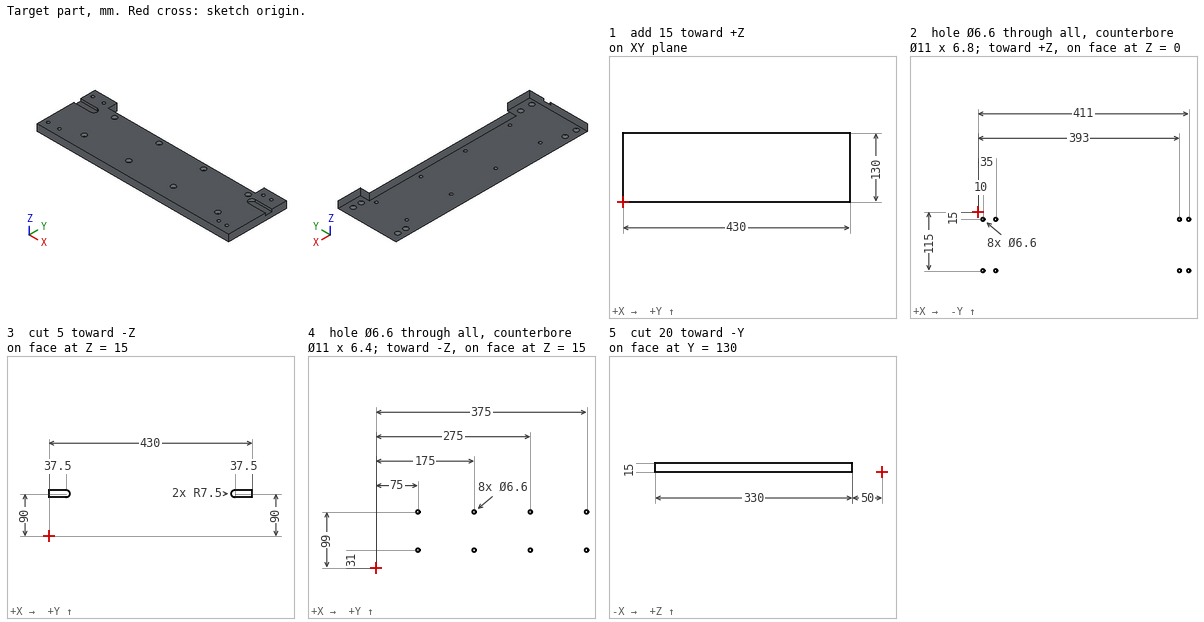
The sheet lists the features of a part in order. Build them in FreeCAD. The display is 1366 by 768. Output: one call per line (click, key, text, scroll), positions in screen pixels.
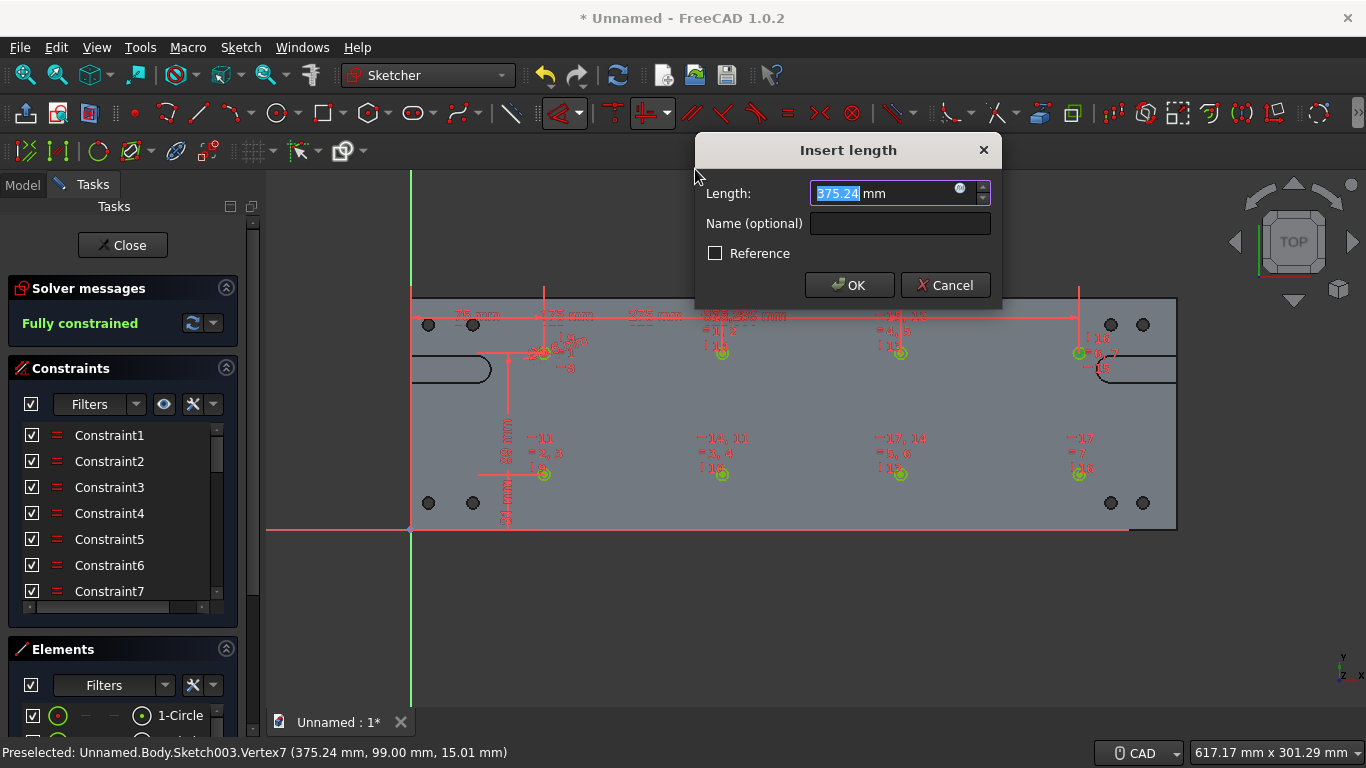
text(375)
key(Return)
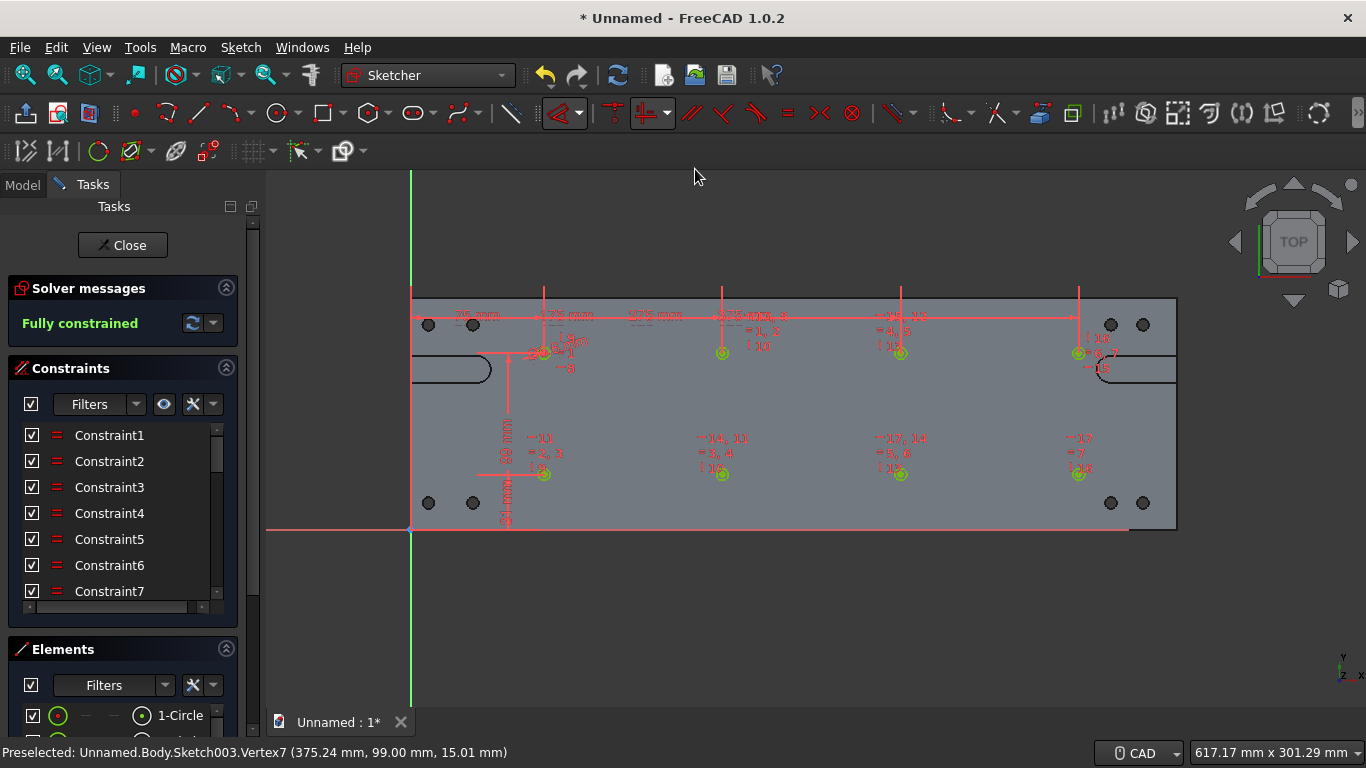
click(123, 245)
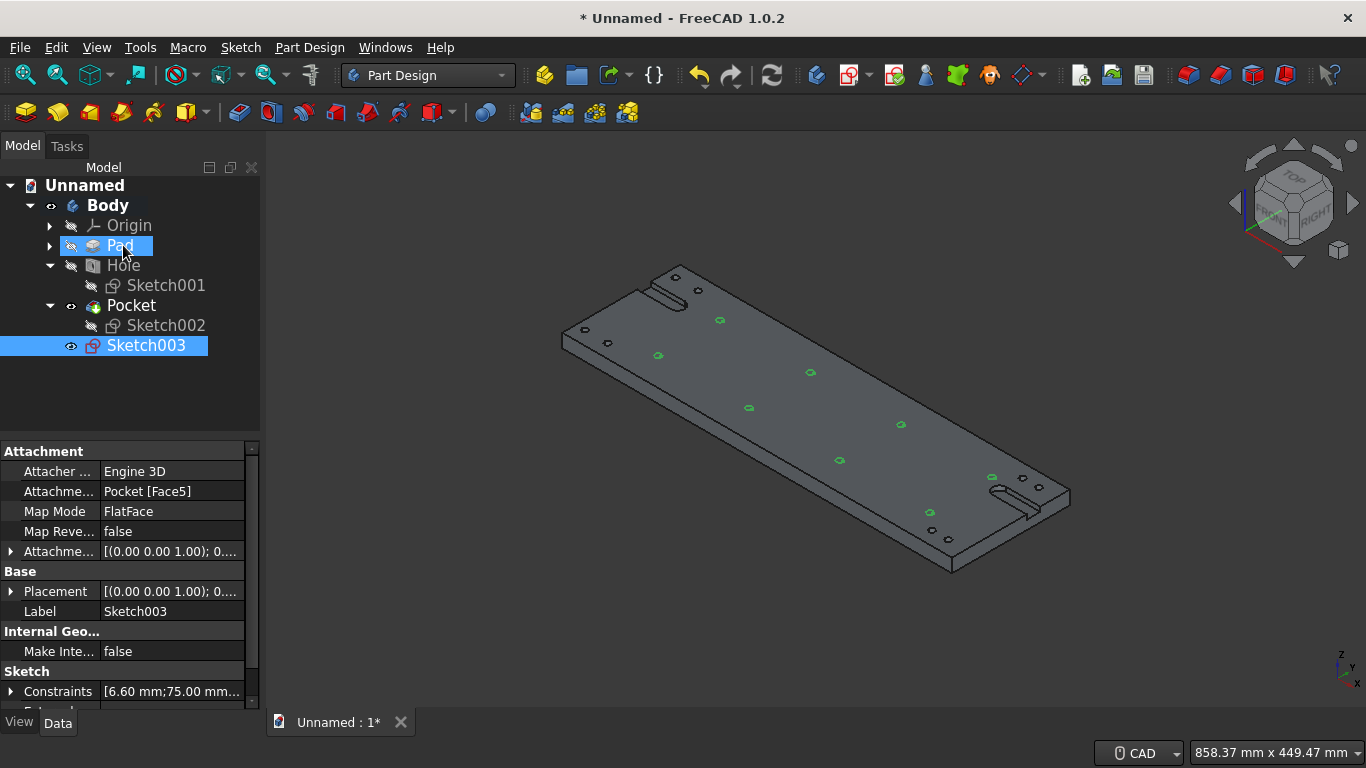
click(272, 112)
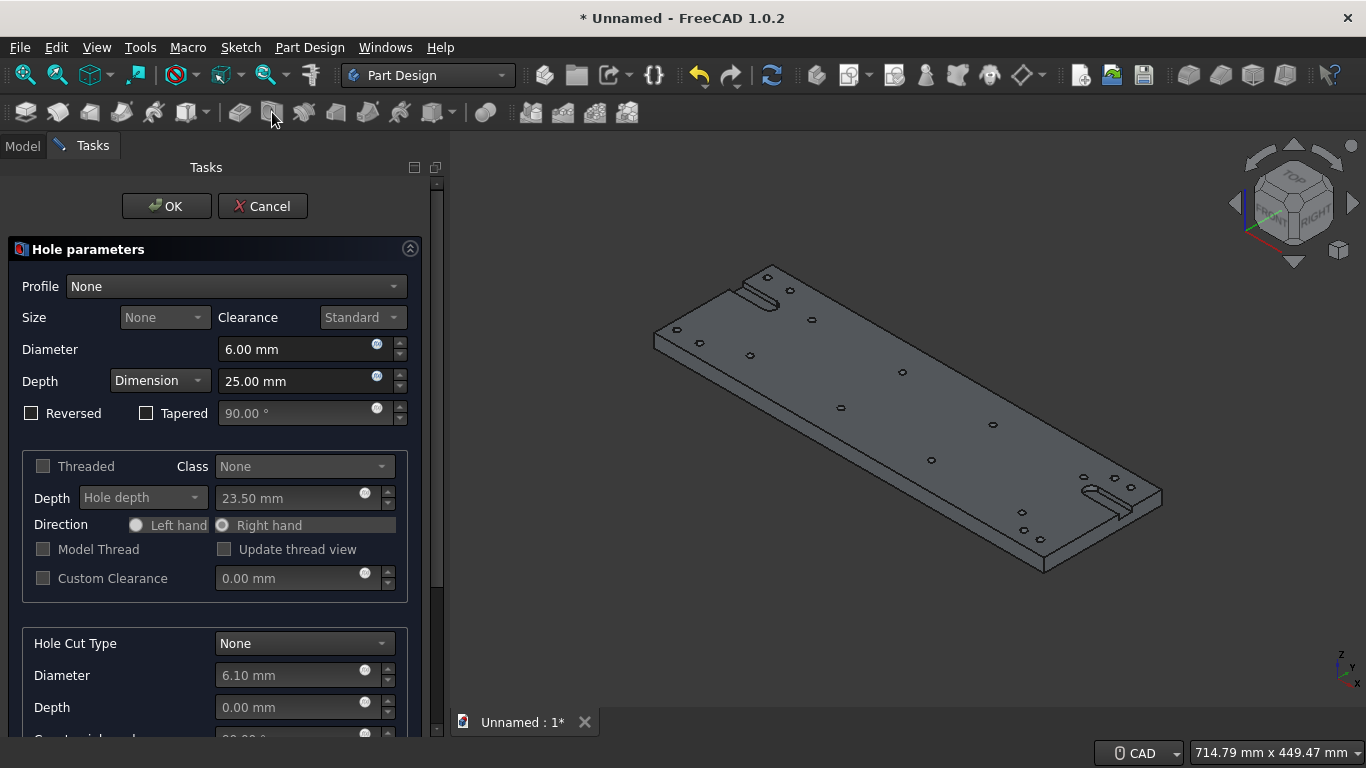
triple_click(305, 349)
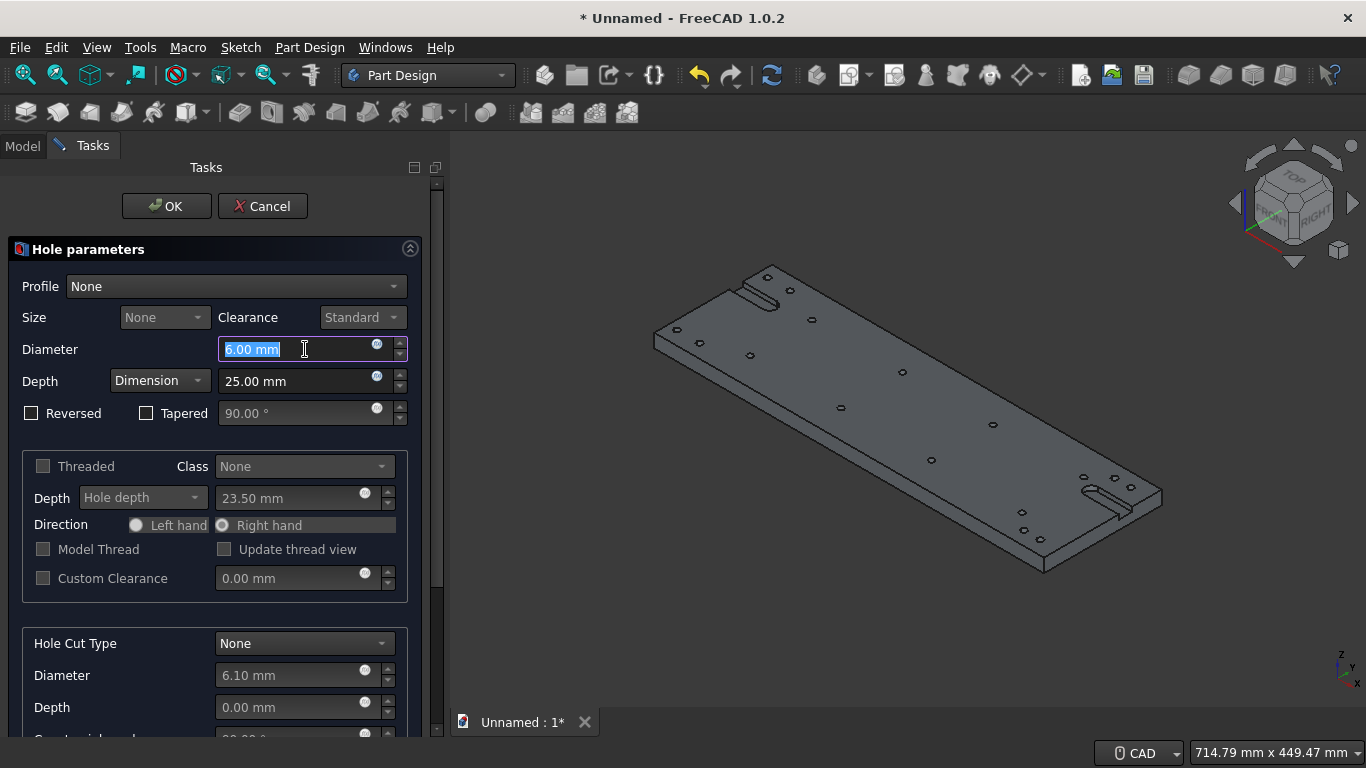
text(6.6)
key(Tab)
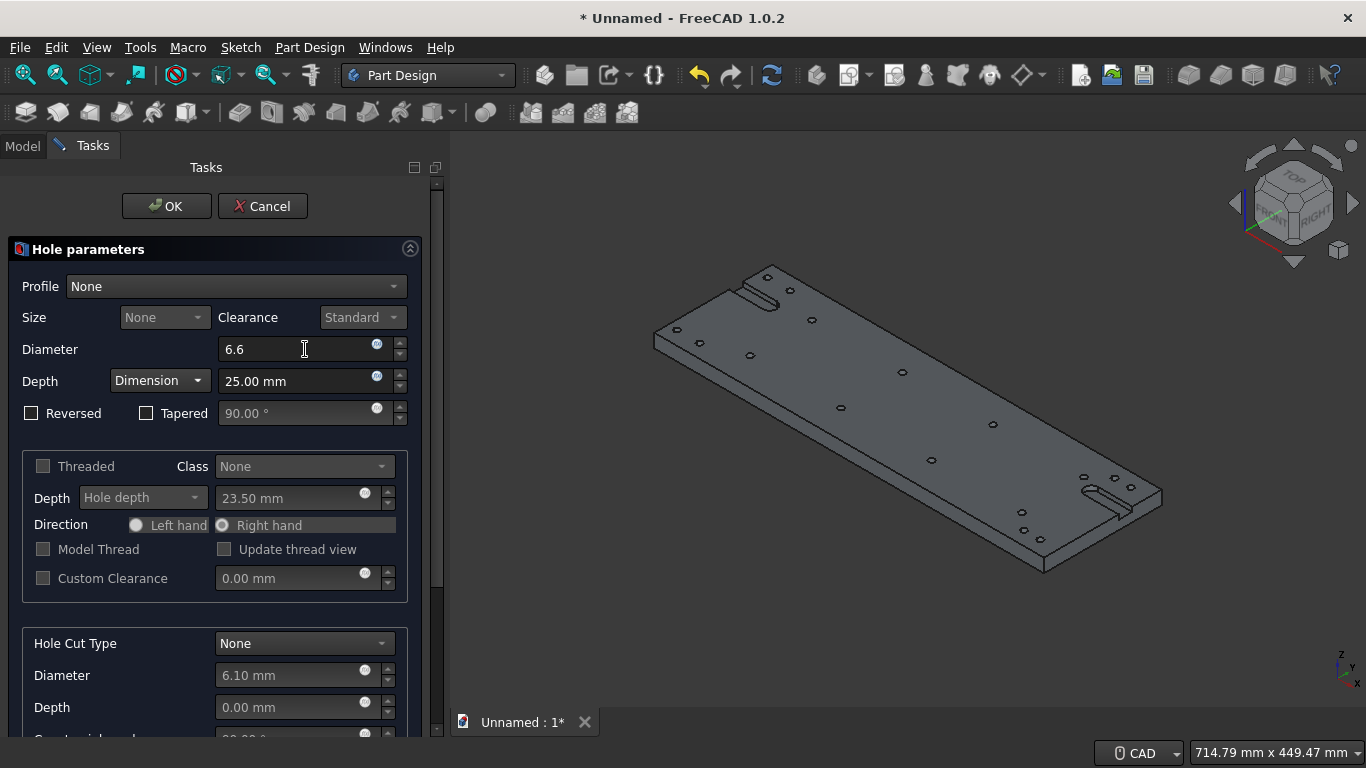
click(161, 380)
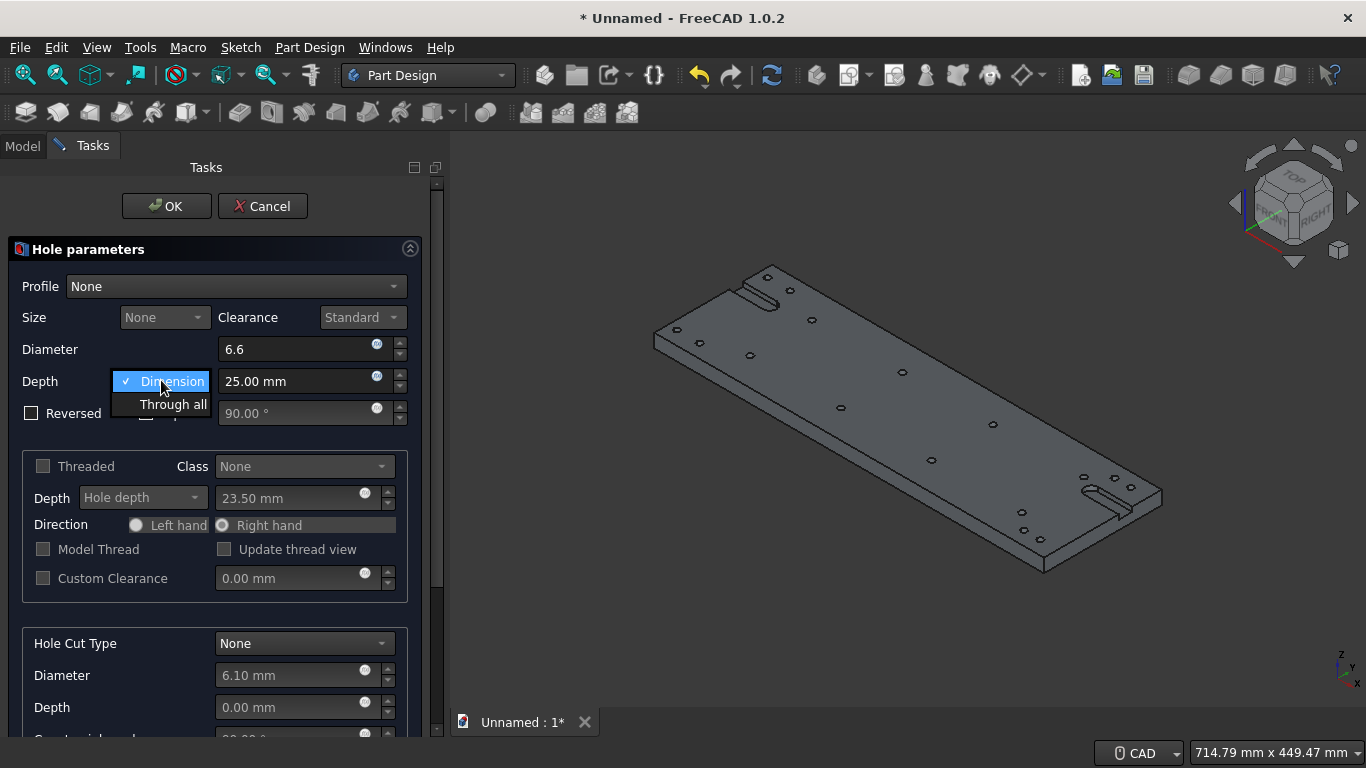
click(160, 404)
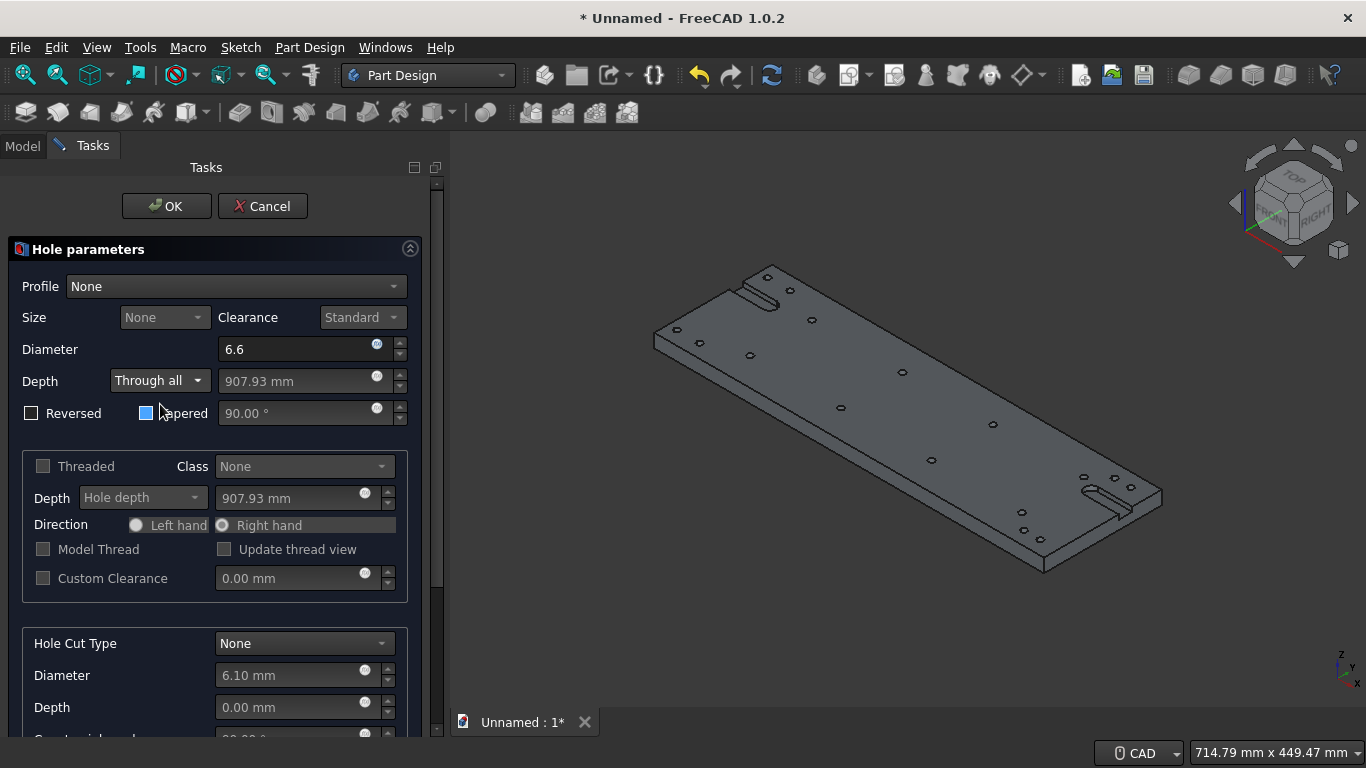
click(306, 644)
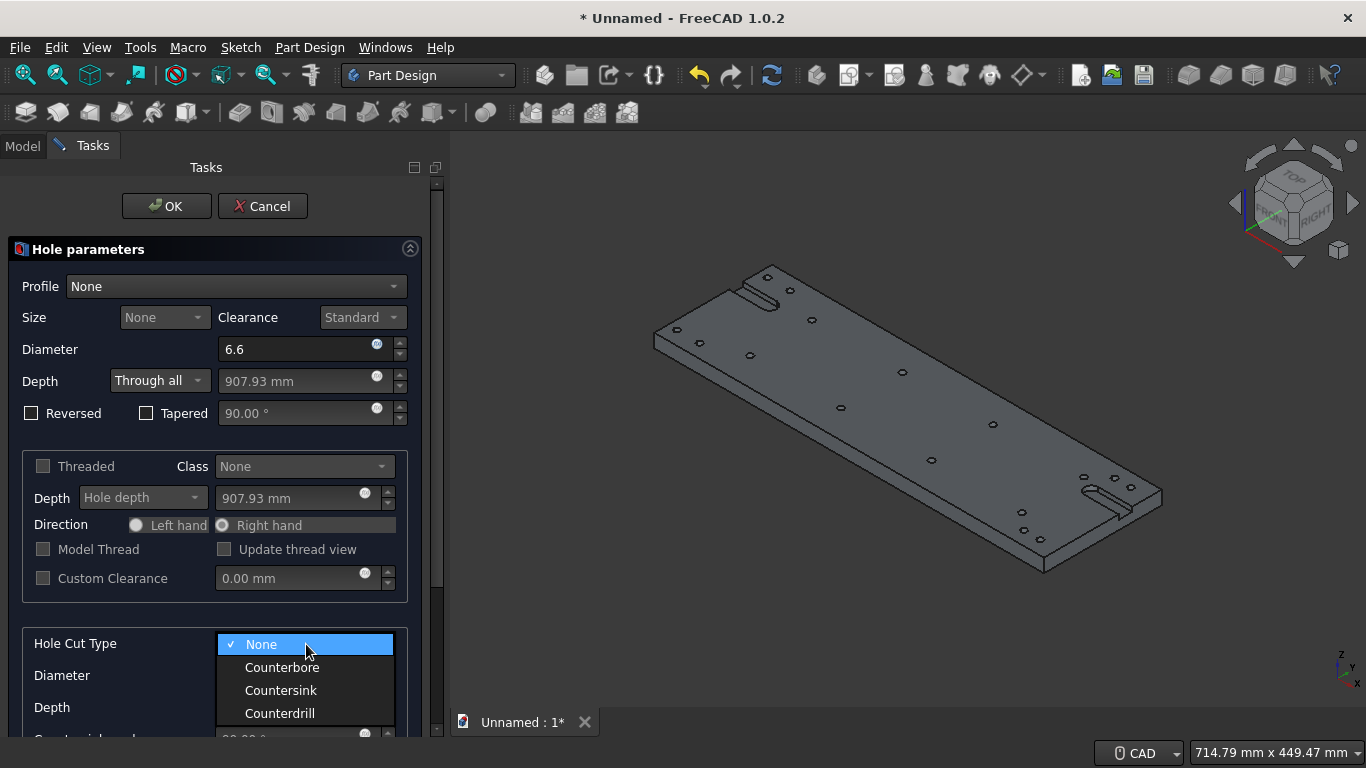
click(304, 668)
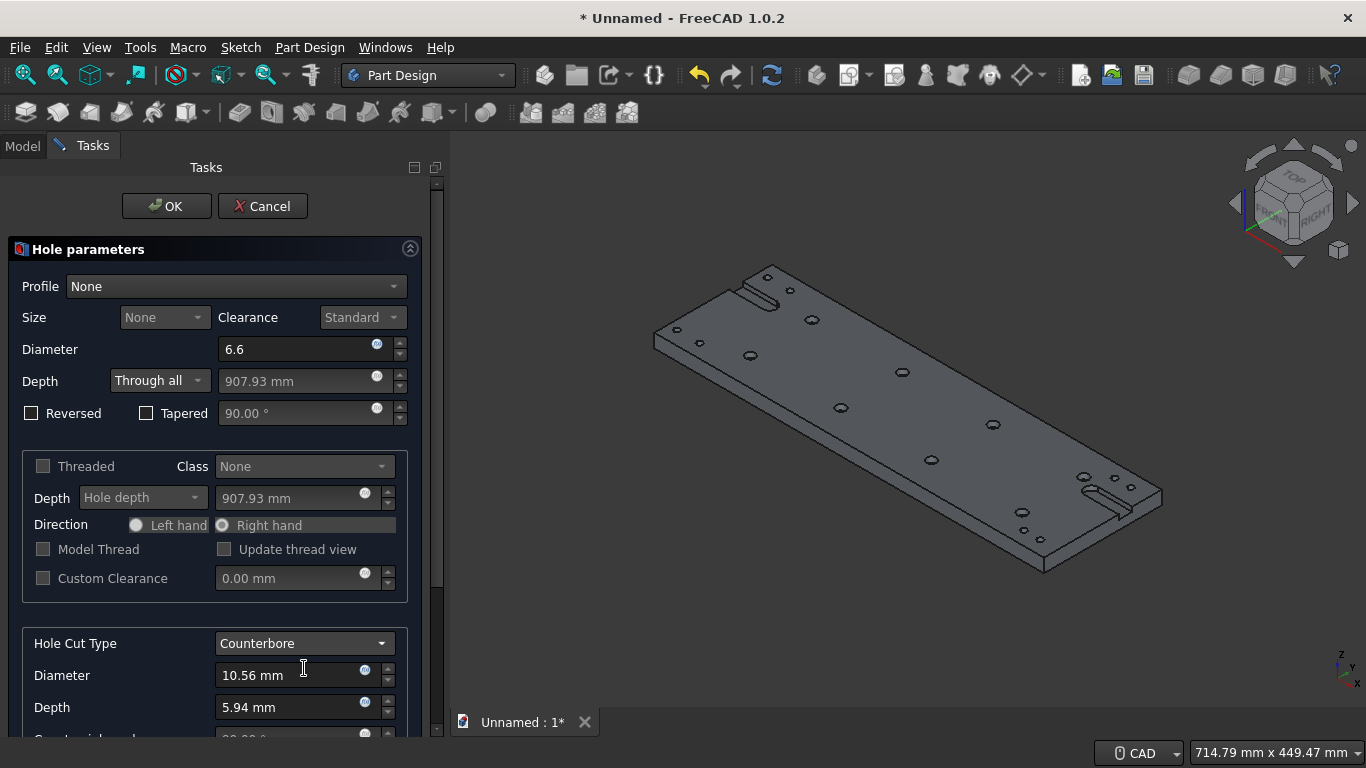
triple_click(298, 675)